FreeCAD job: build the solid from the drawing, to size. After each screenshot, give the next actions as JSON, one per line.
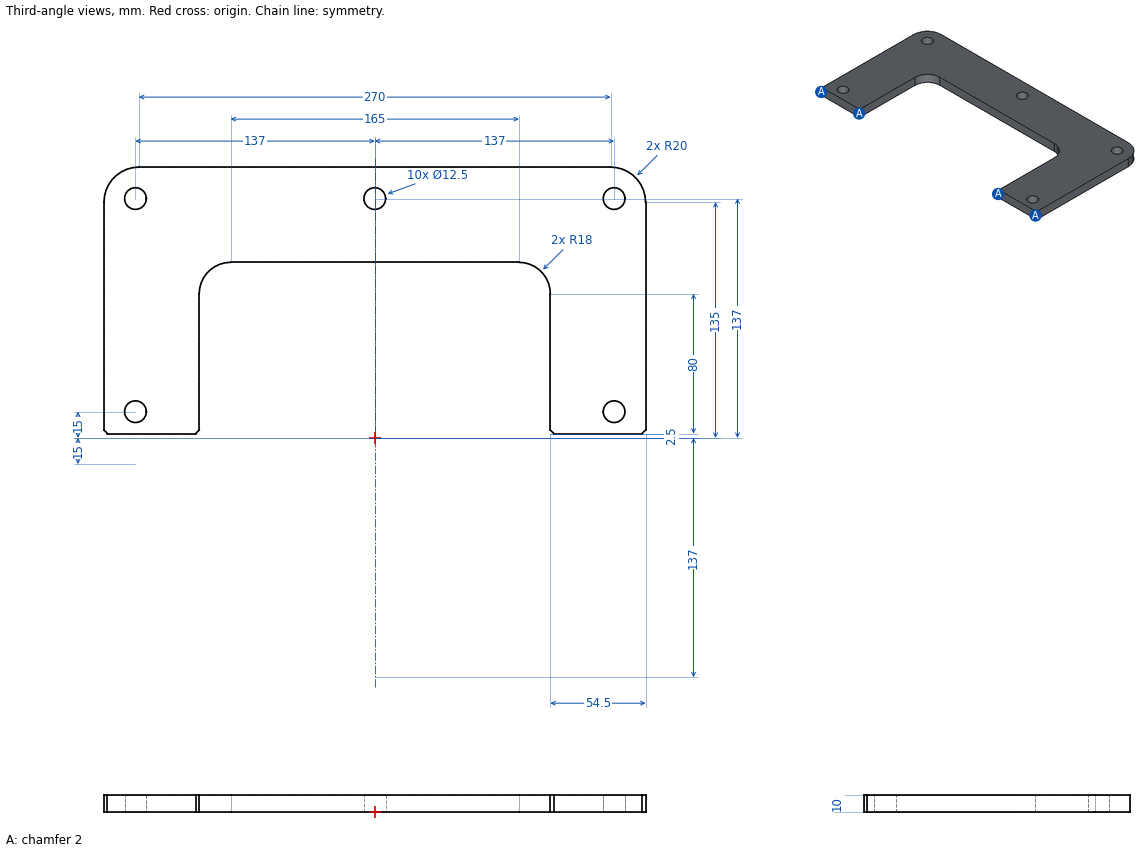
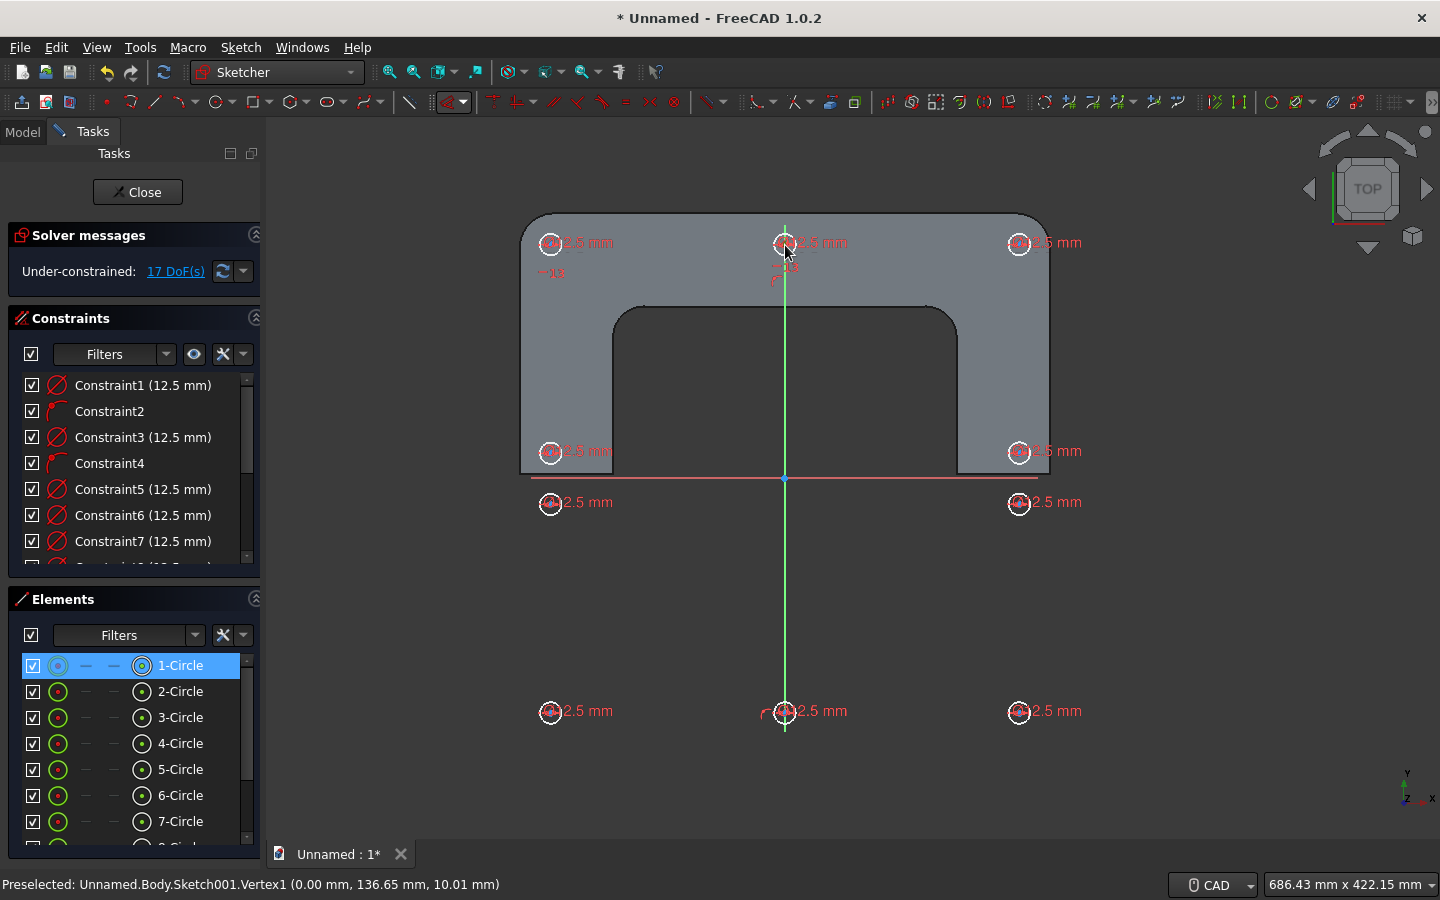
{"action": "left_click", "coordinate": [1019, 245]}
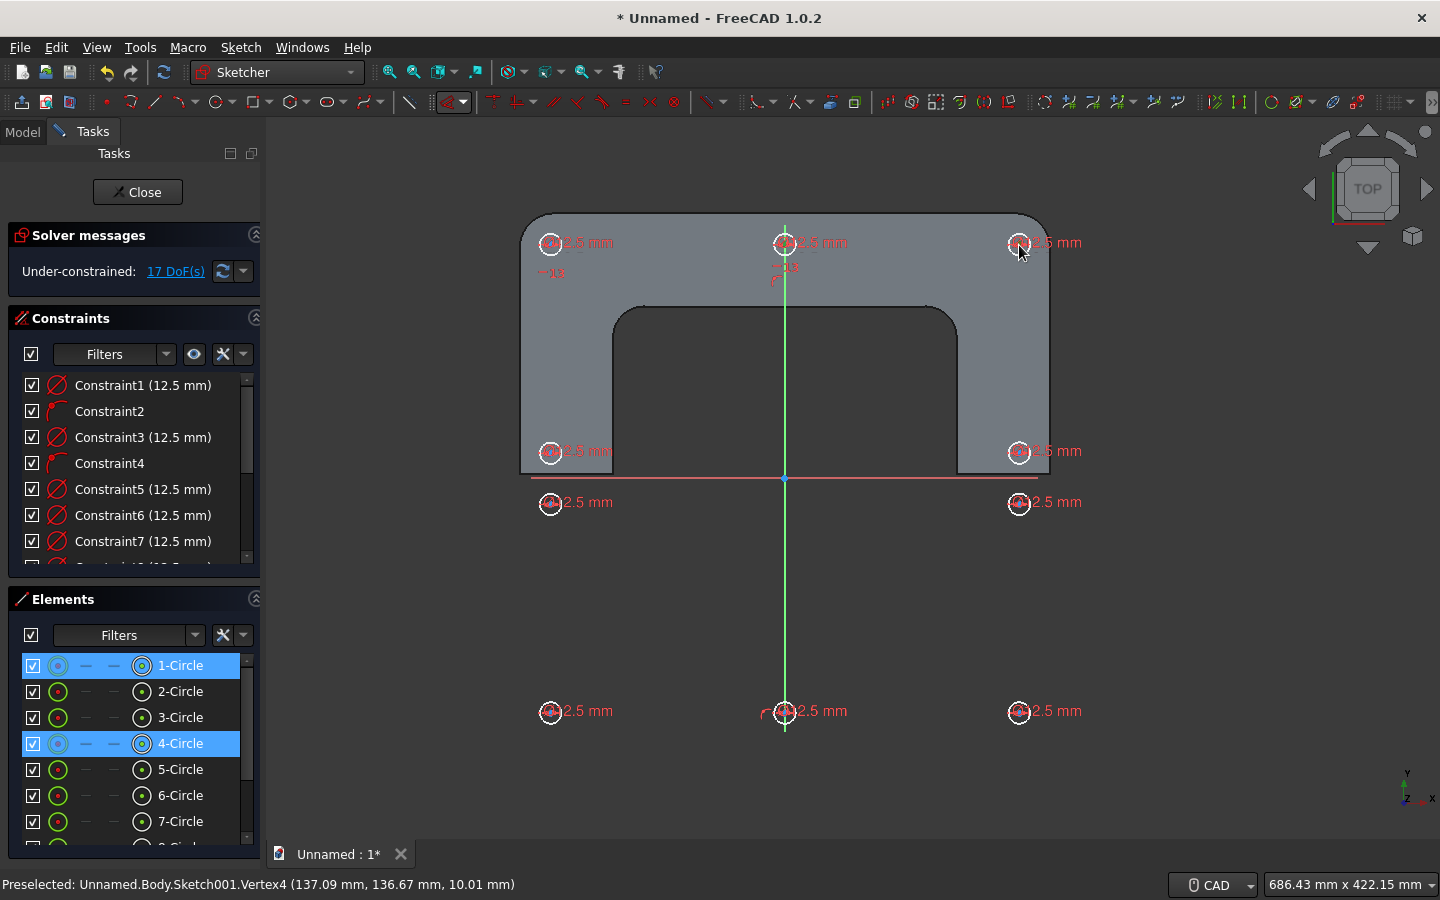
{"action": "key", "text": "h"}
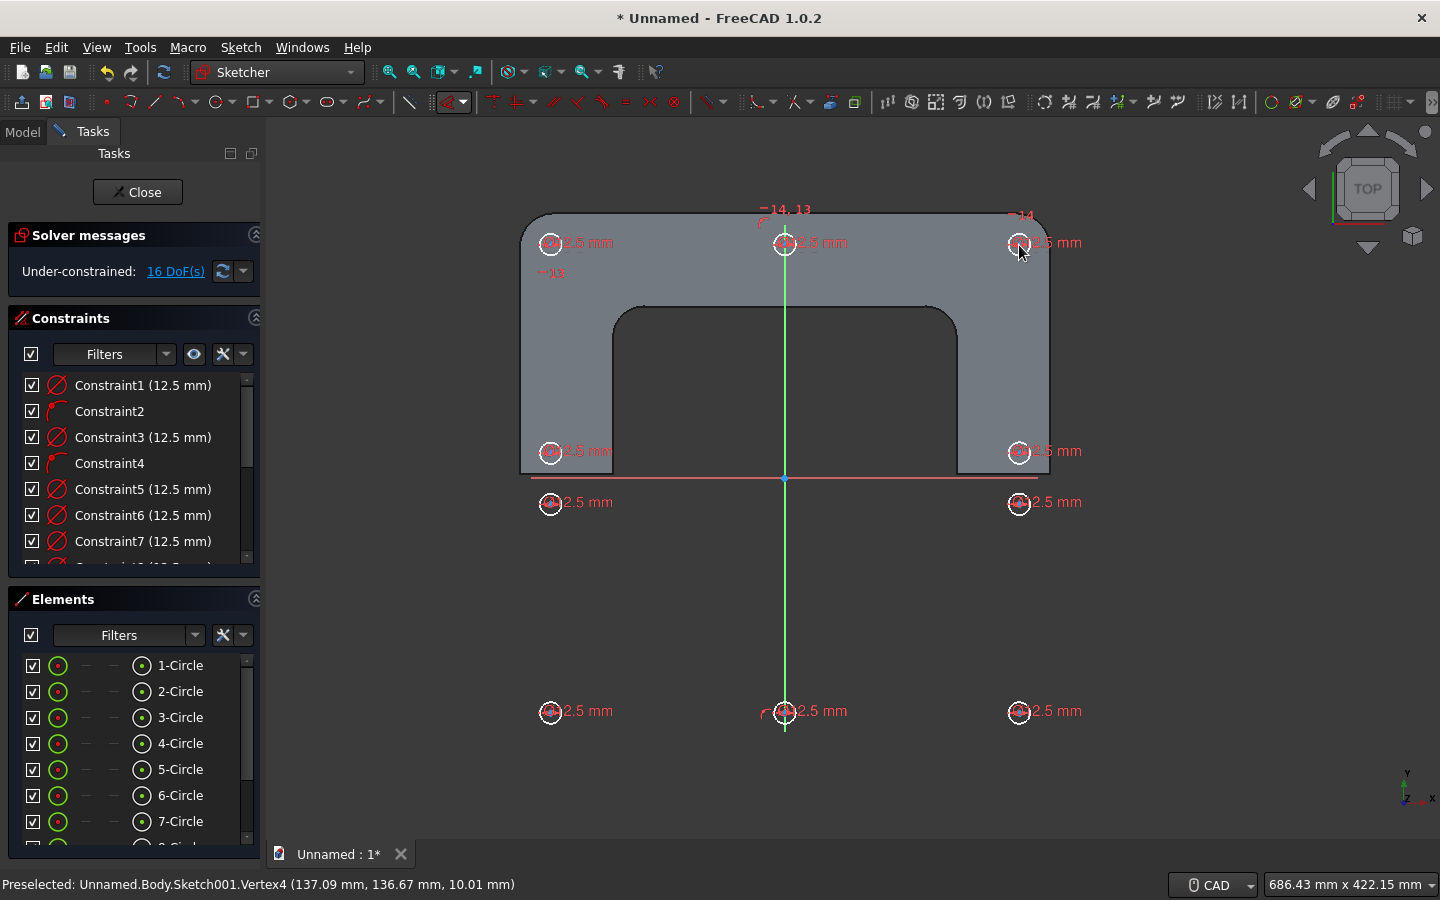
{"action": "left_click", "coordinate": [551, 245]}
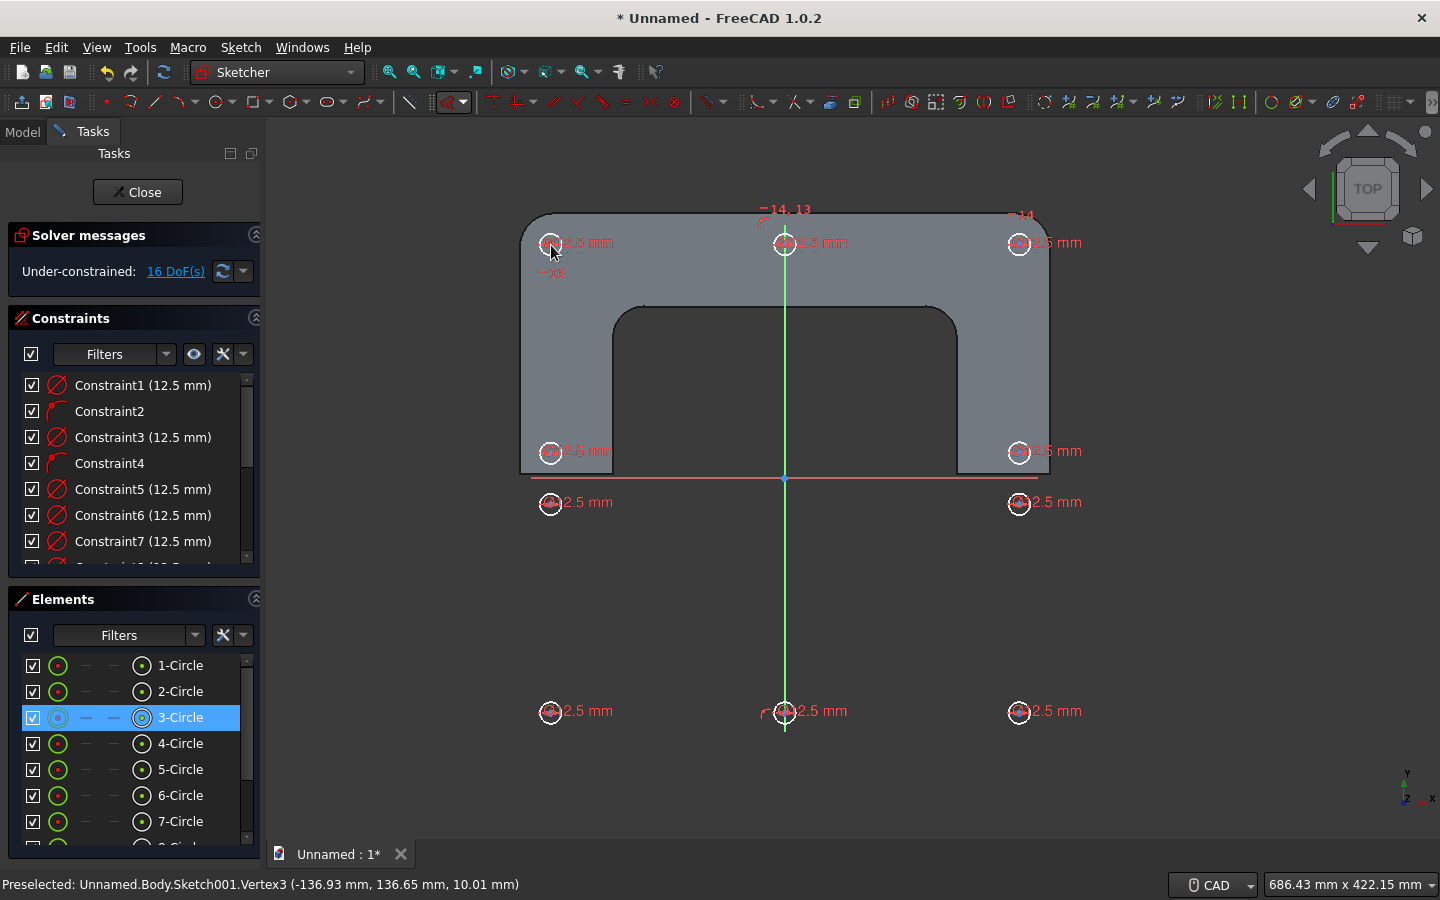
{"action": "left_click", "coordinate": [551, 713]}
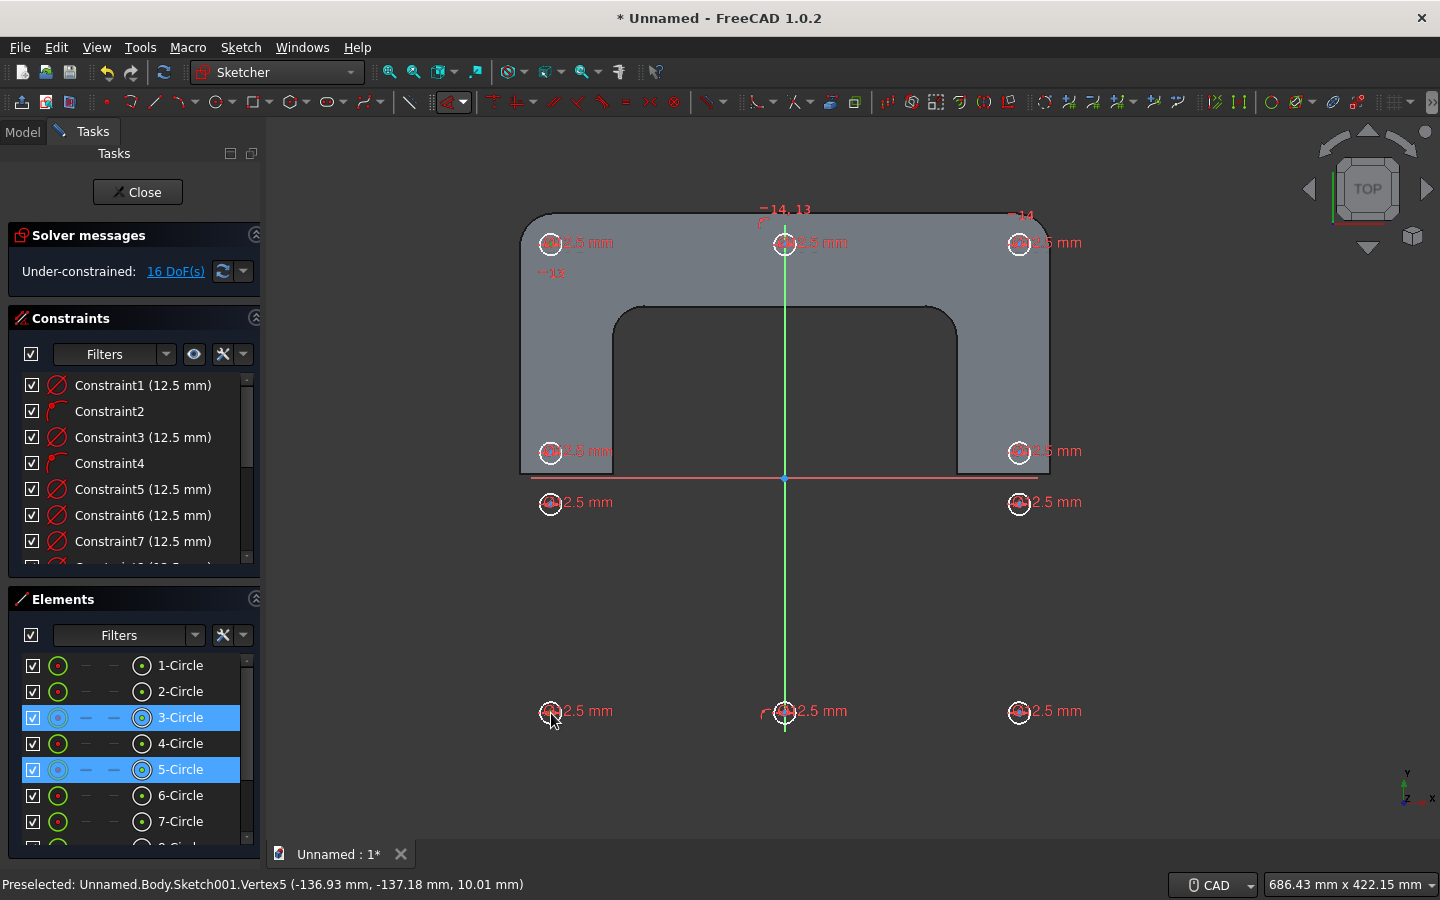
{"action": "key", "text": "v"}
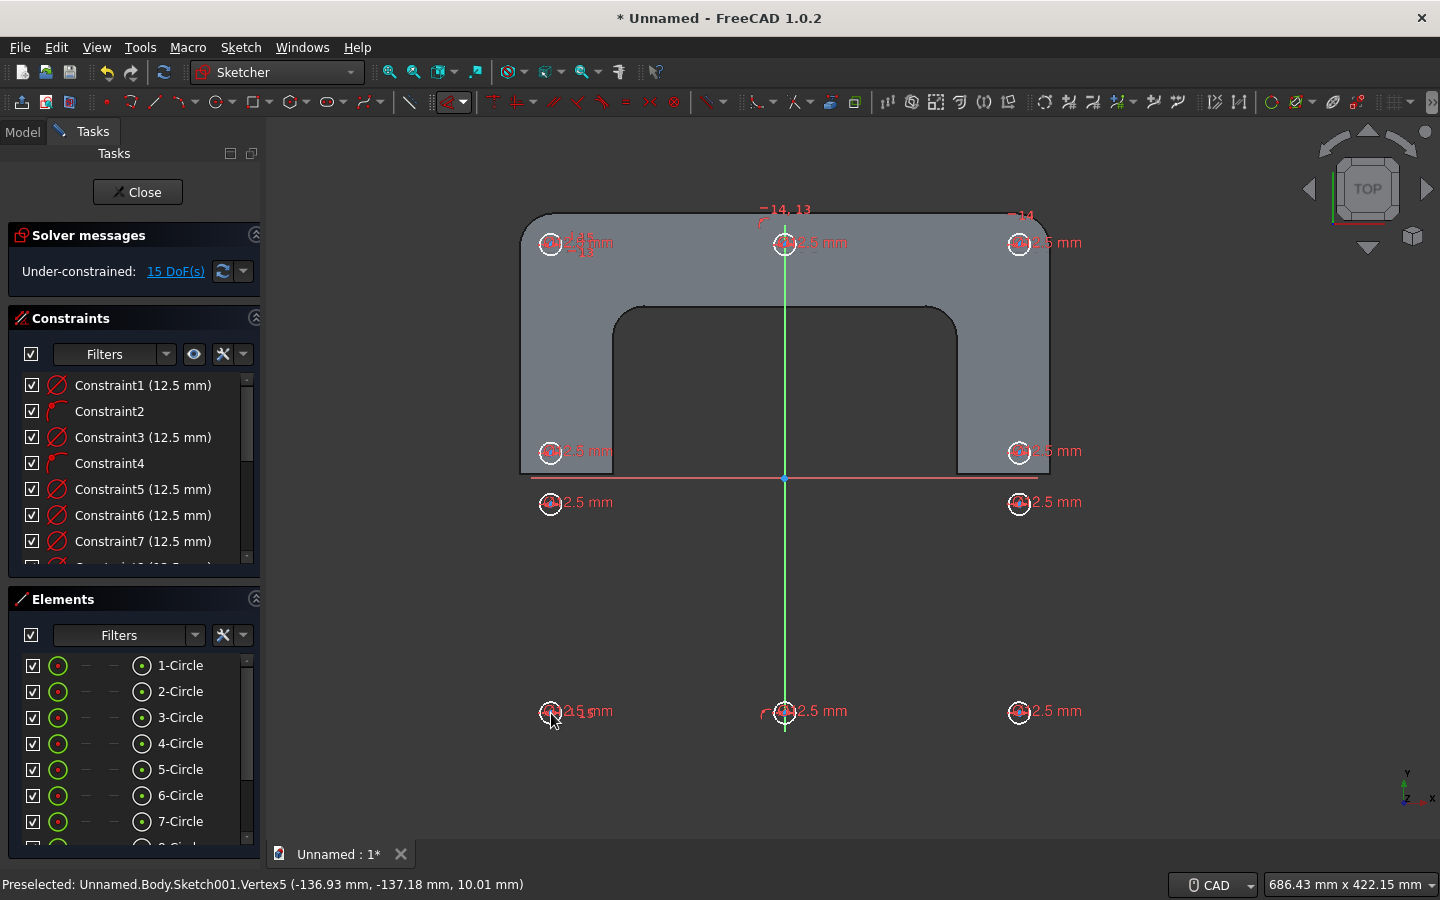
{"action": "left_click", "coordinate": [785, 713]}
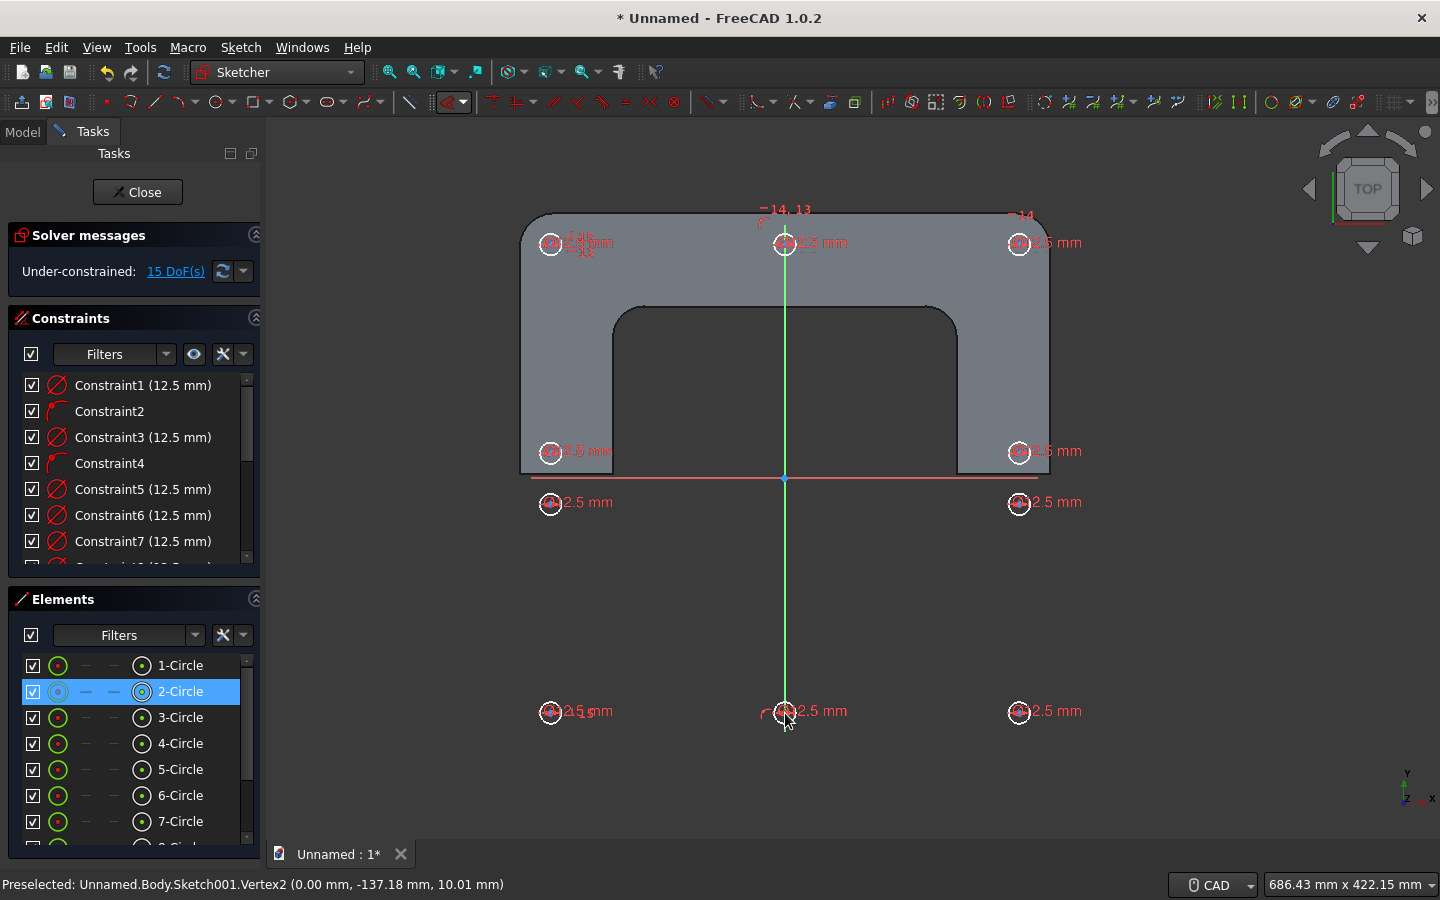
{"action": "left_click", "coordinate": [551, 713]}